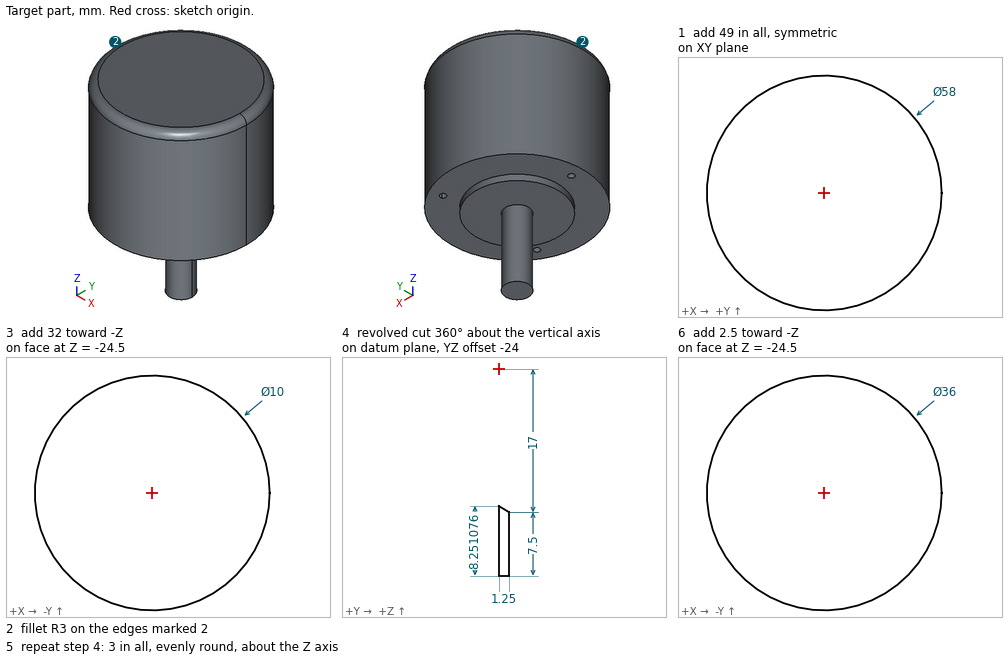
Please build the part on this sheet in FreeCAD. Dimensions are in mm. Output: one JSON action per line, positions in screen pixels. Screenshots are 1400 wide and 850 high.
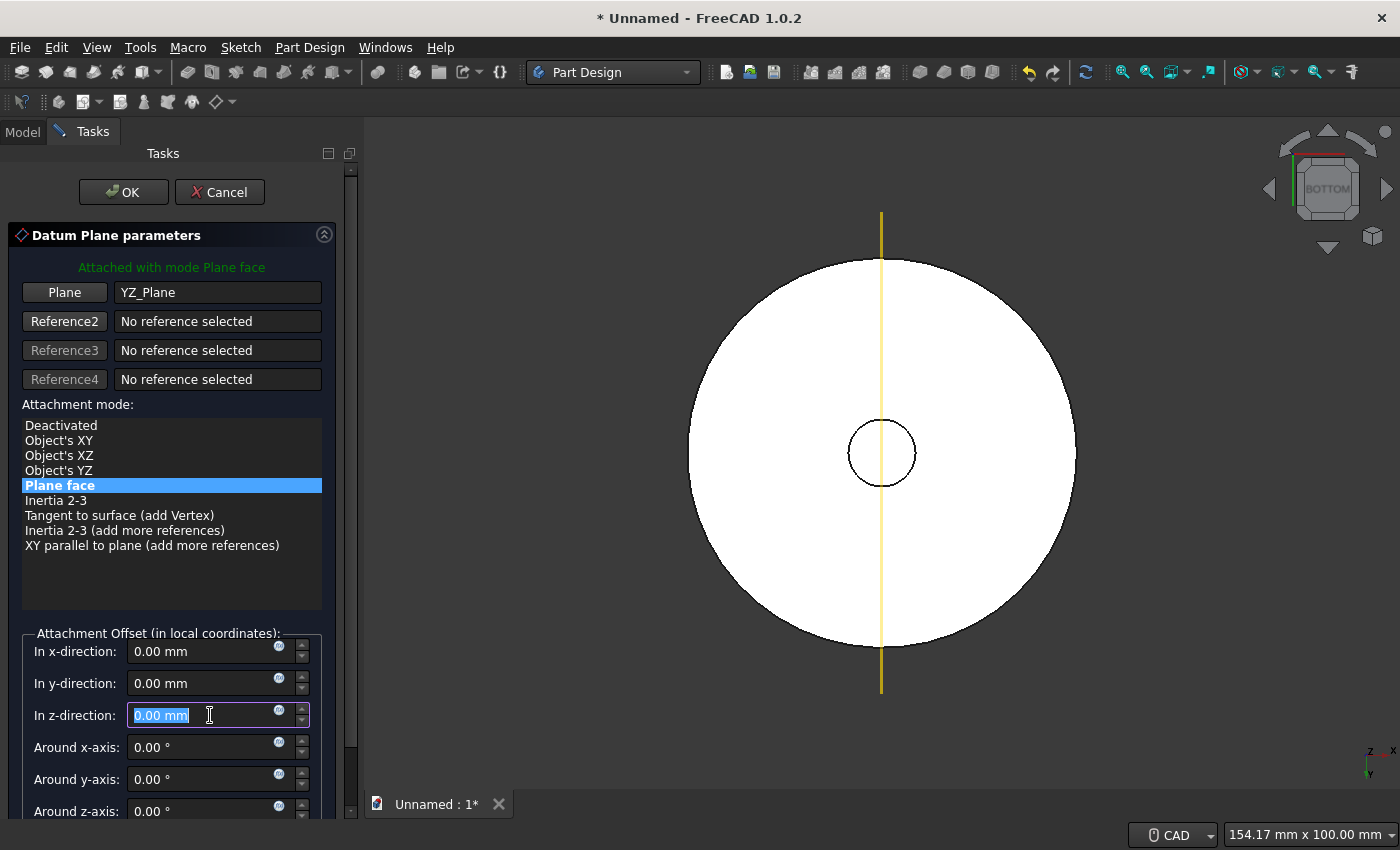
{"action": "type", "text": "-24"}
{"action": "key", "text": "Tab"}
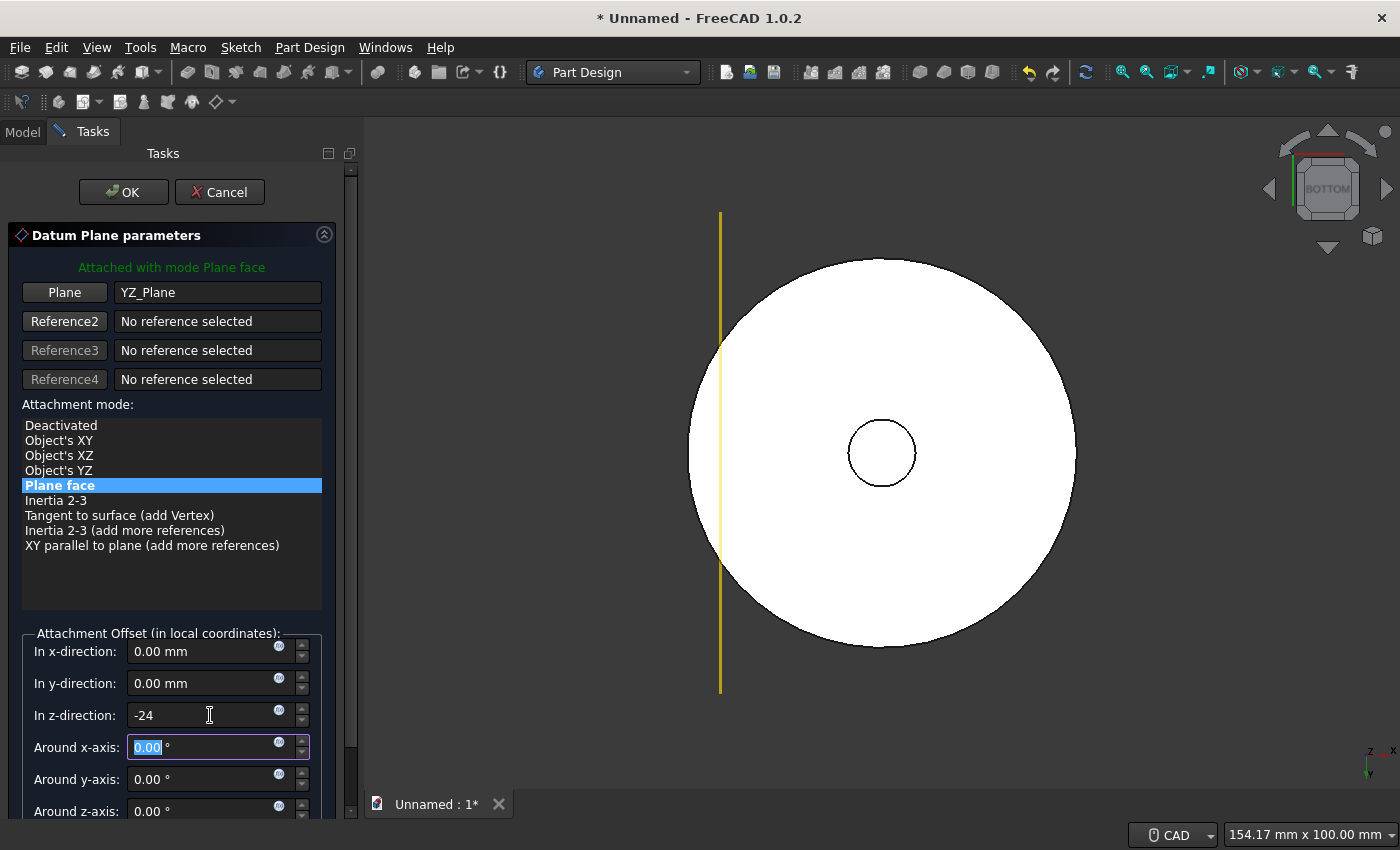
{"action": "left_click", "coordinate": [124, 192]}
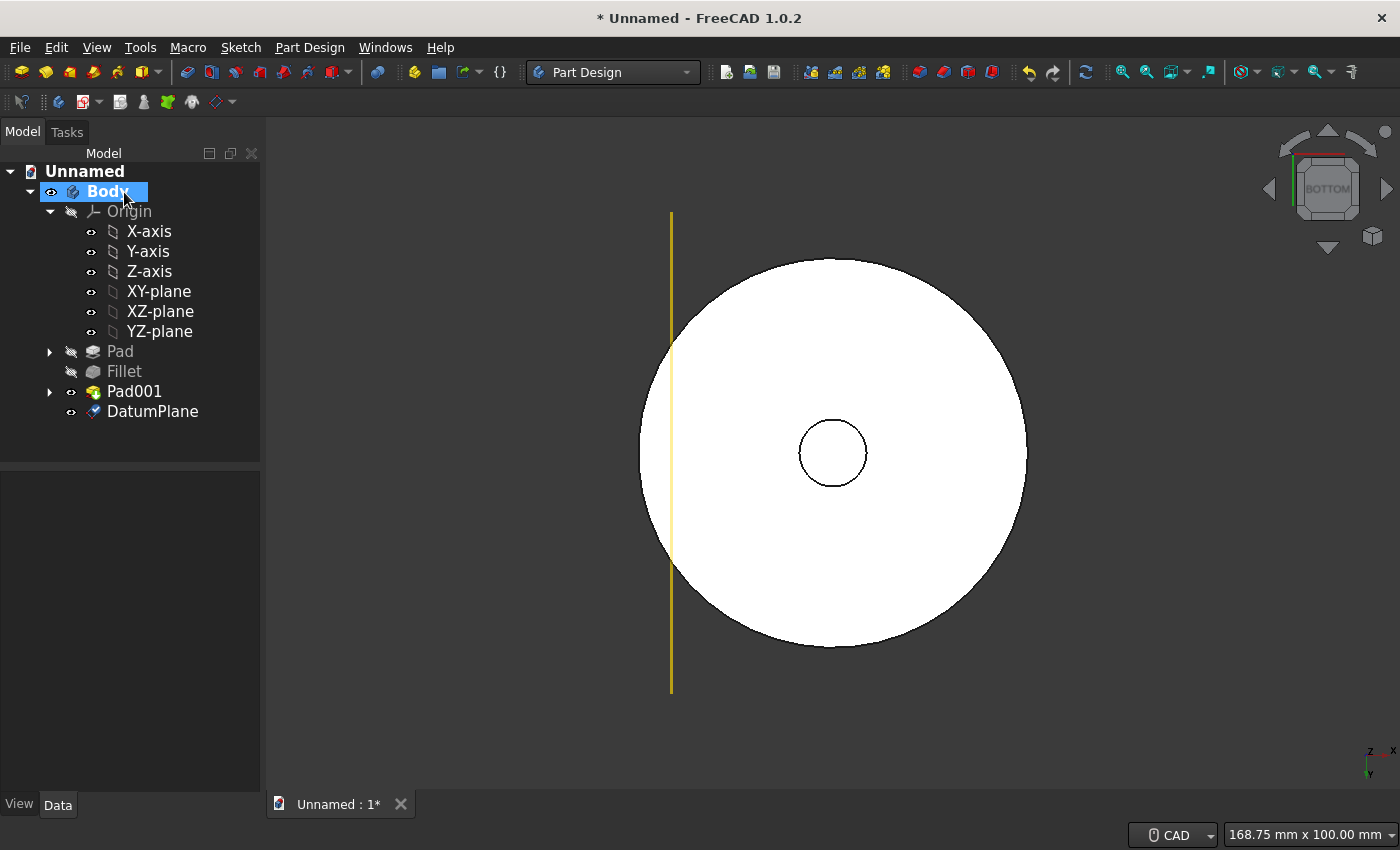
{"action": "left_click", "coordinate": [116, 412]}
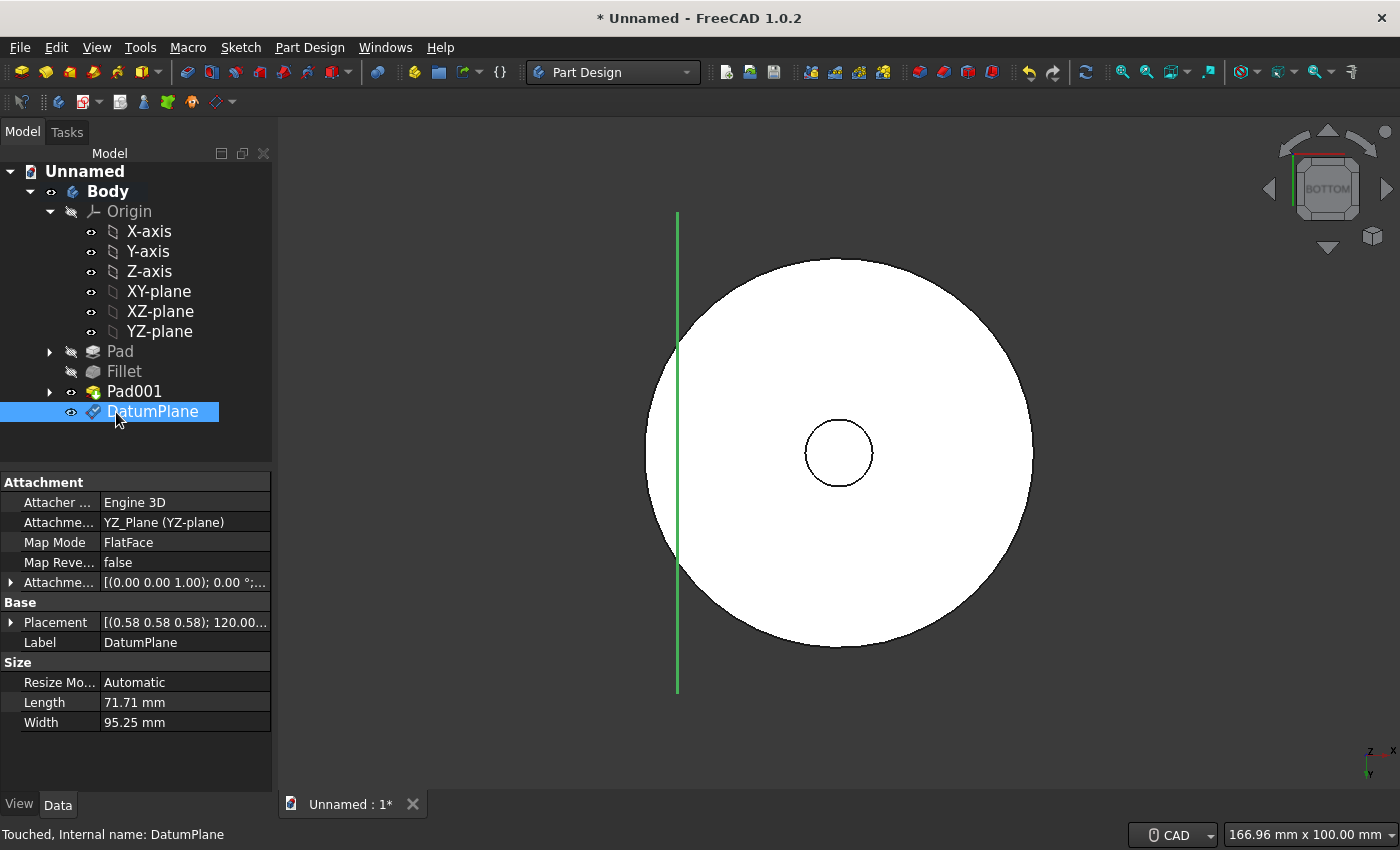
{"action": "left_click", "coordinate": [84, 102]}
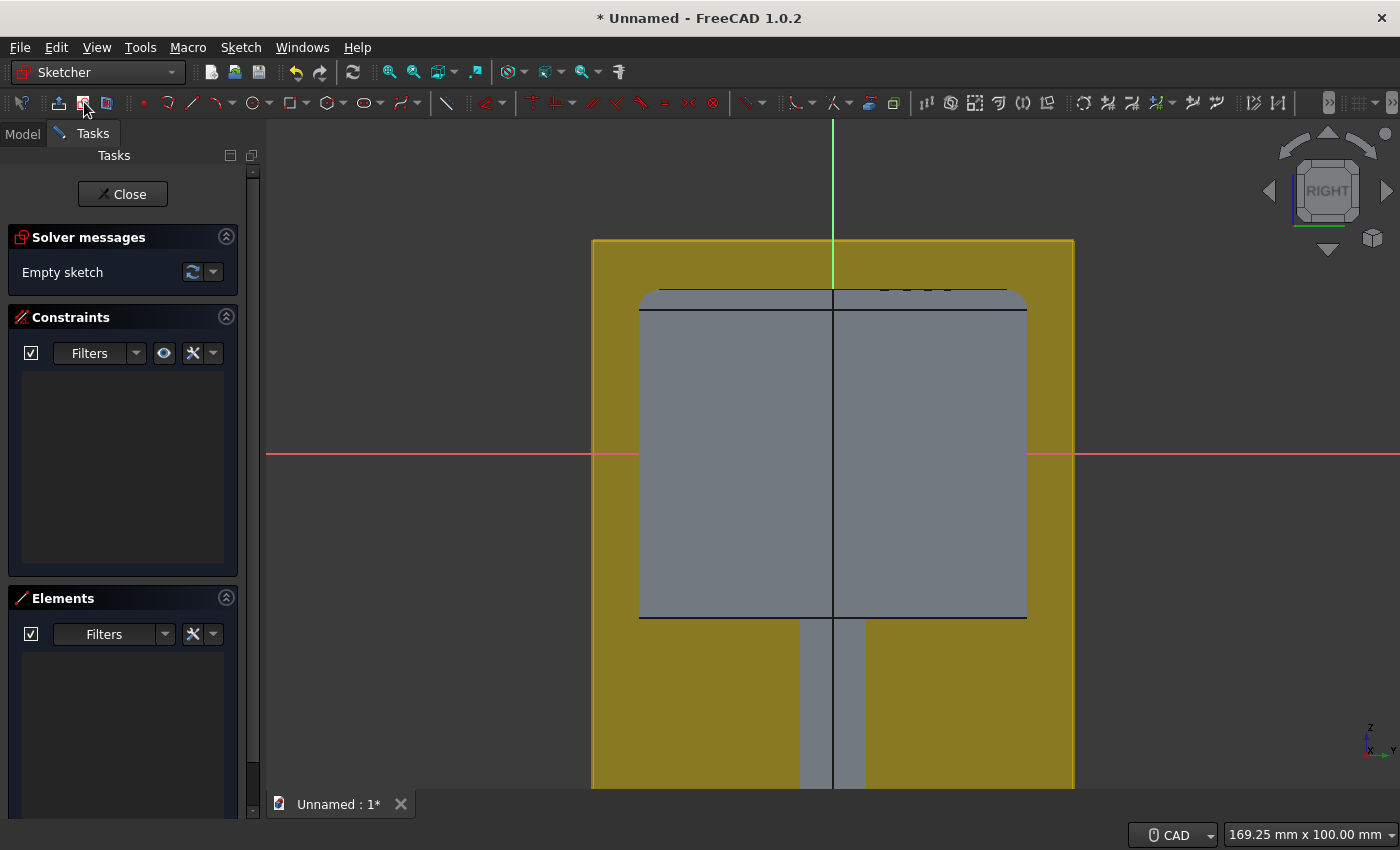
{"action": "left_click", "coordinate": [108, 104]}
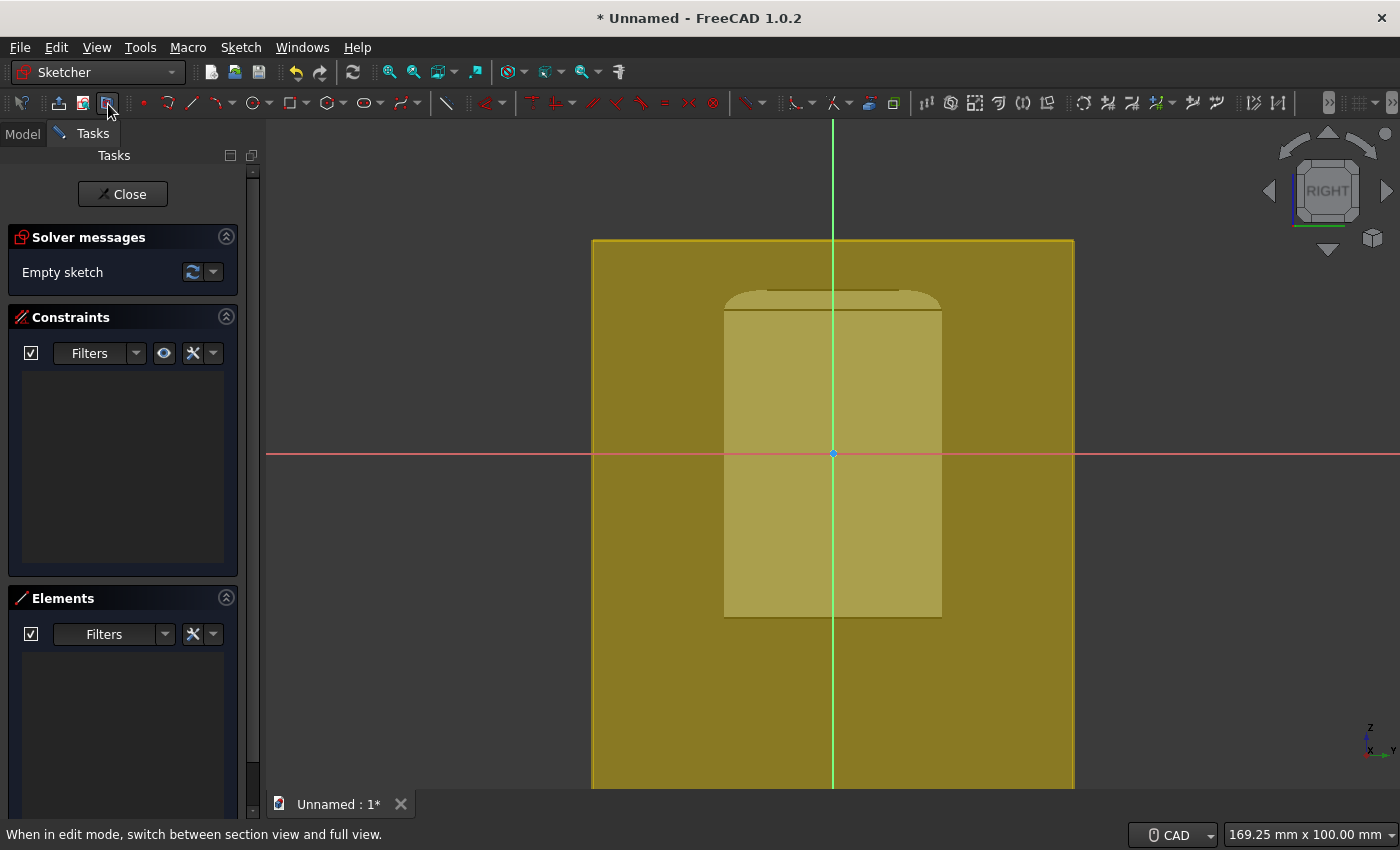
{"action": "scroll", "coordinate": [849, 612], "scroll_direction": "up", "scroll_amount": 10}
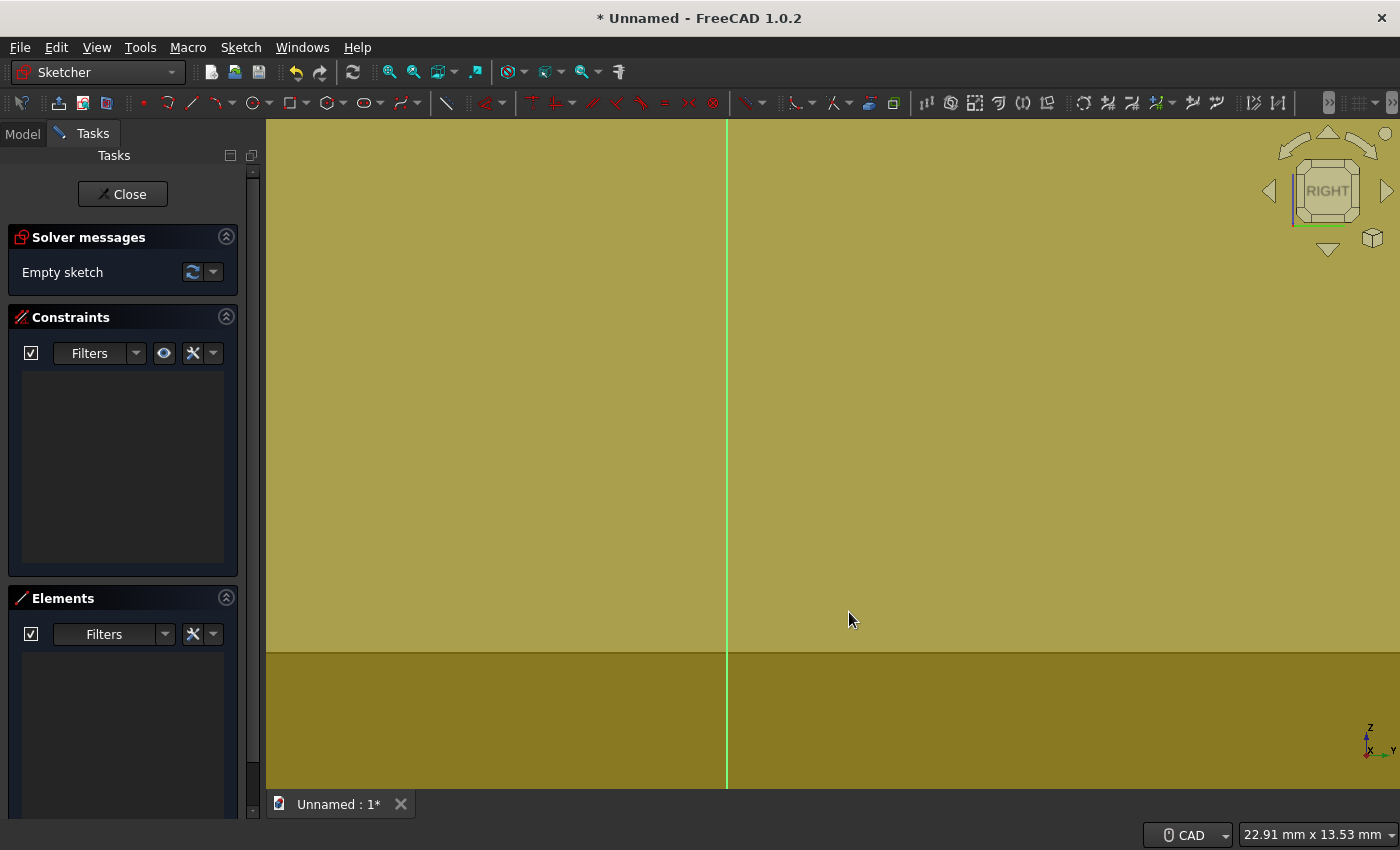
{"action": "left_click", "coordinate": [168, 104]}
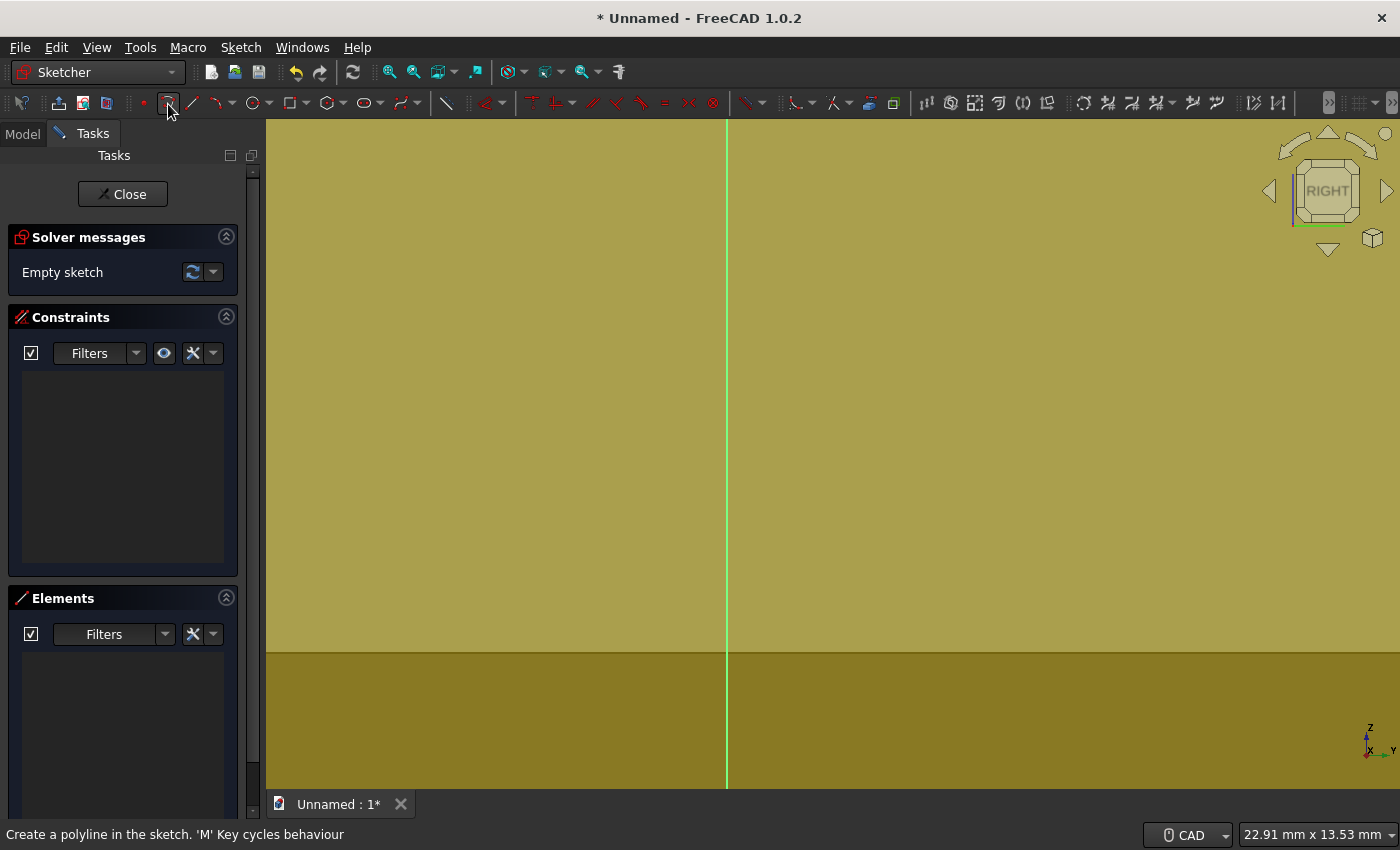
{"action": "left_click", "coordinate": [727, 244]}
{"action": "left_click", "coordinate": [736, 653]}
{"action": "left_click", "coordinate": [789, 653]}
{"action": "left_click", "coordinate": [789, 281]}
{"action": "left_click", "coordinate": [727, 245]}
{"action": "key", "text": "Escape"}
{"action": "key", "text": "Escape"}